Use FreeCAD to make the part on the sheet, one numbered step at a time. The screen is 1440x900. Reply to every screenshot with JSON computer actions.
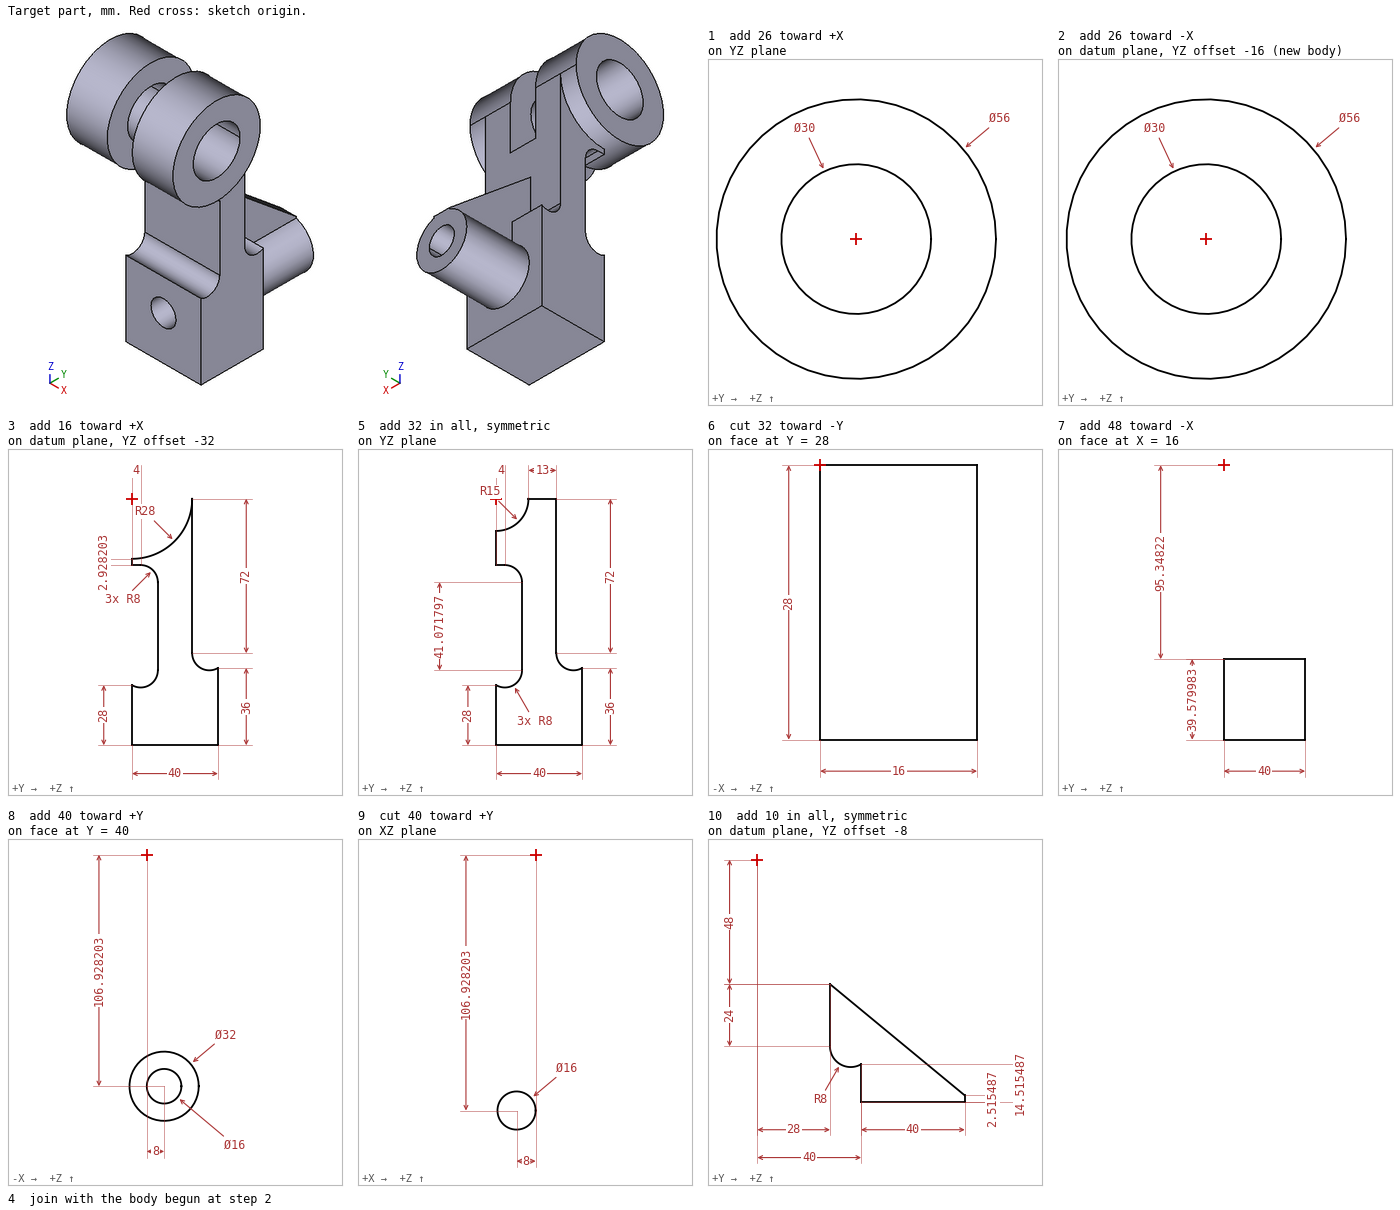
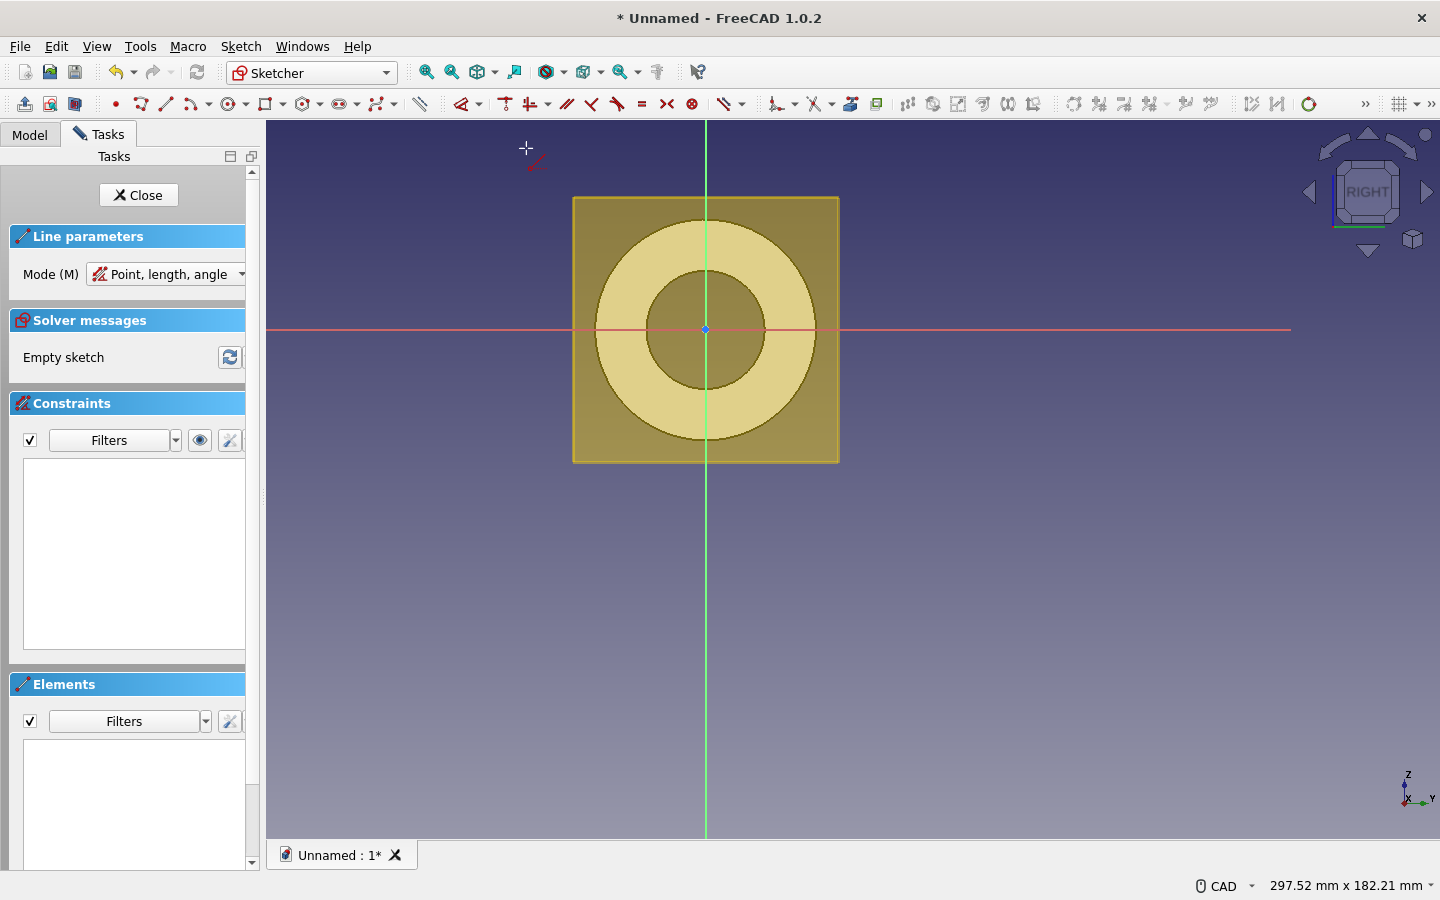
{"action": "left_click", "coordinate": [816, 614]}
{"action": "left_click", "coordinate": [816, 330]}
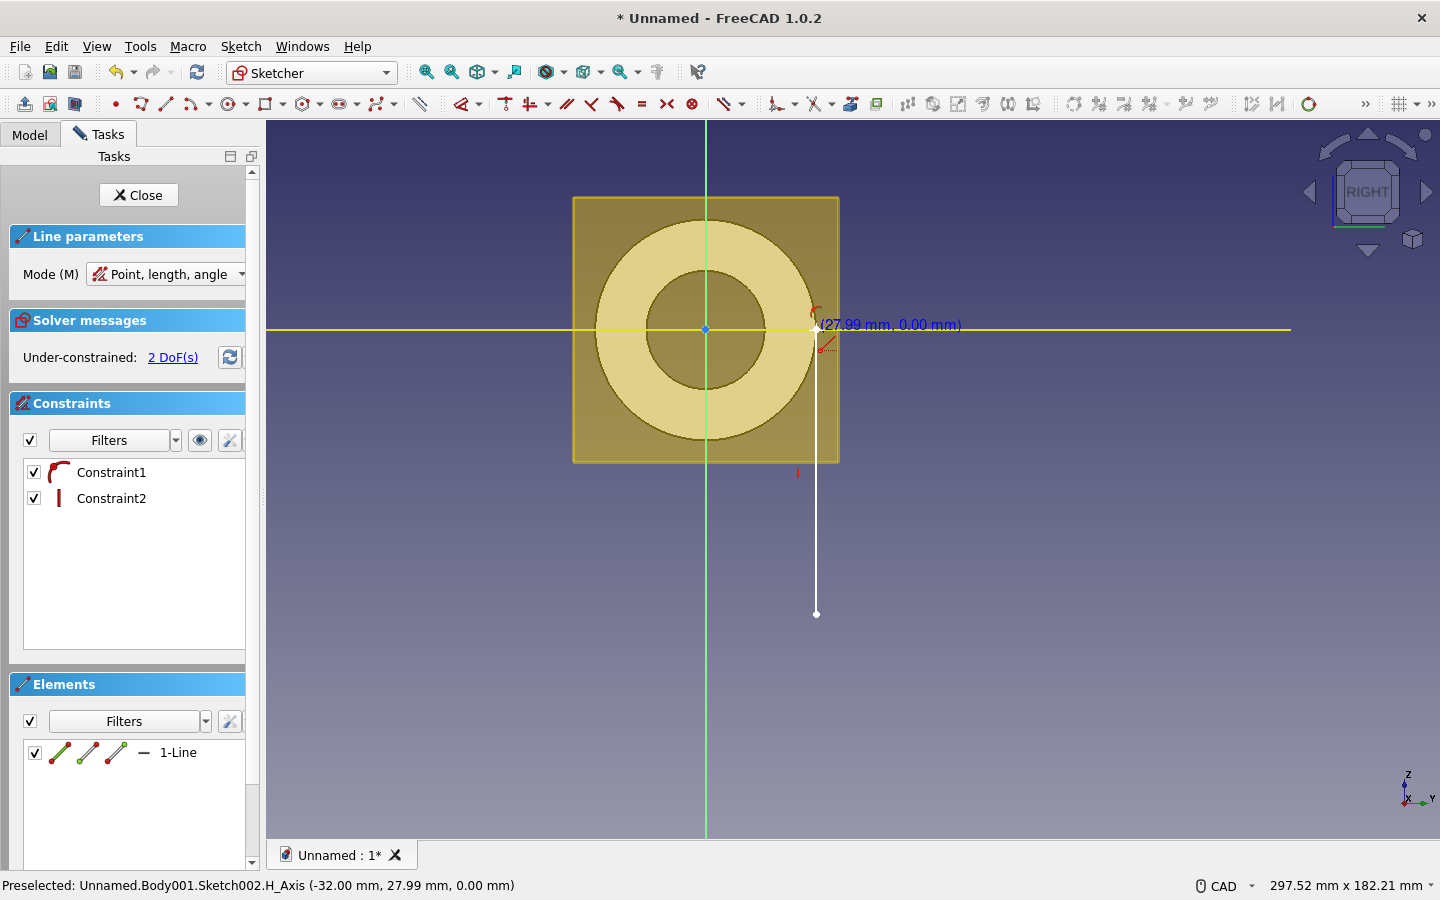
{"action": "left_click", "coordinate": [141, 104]}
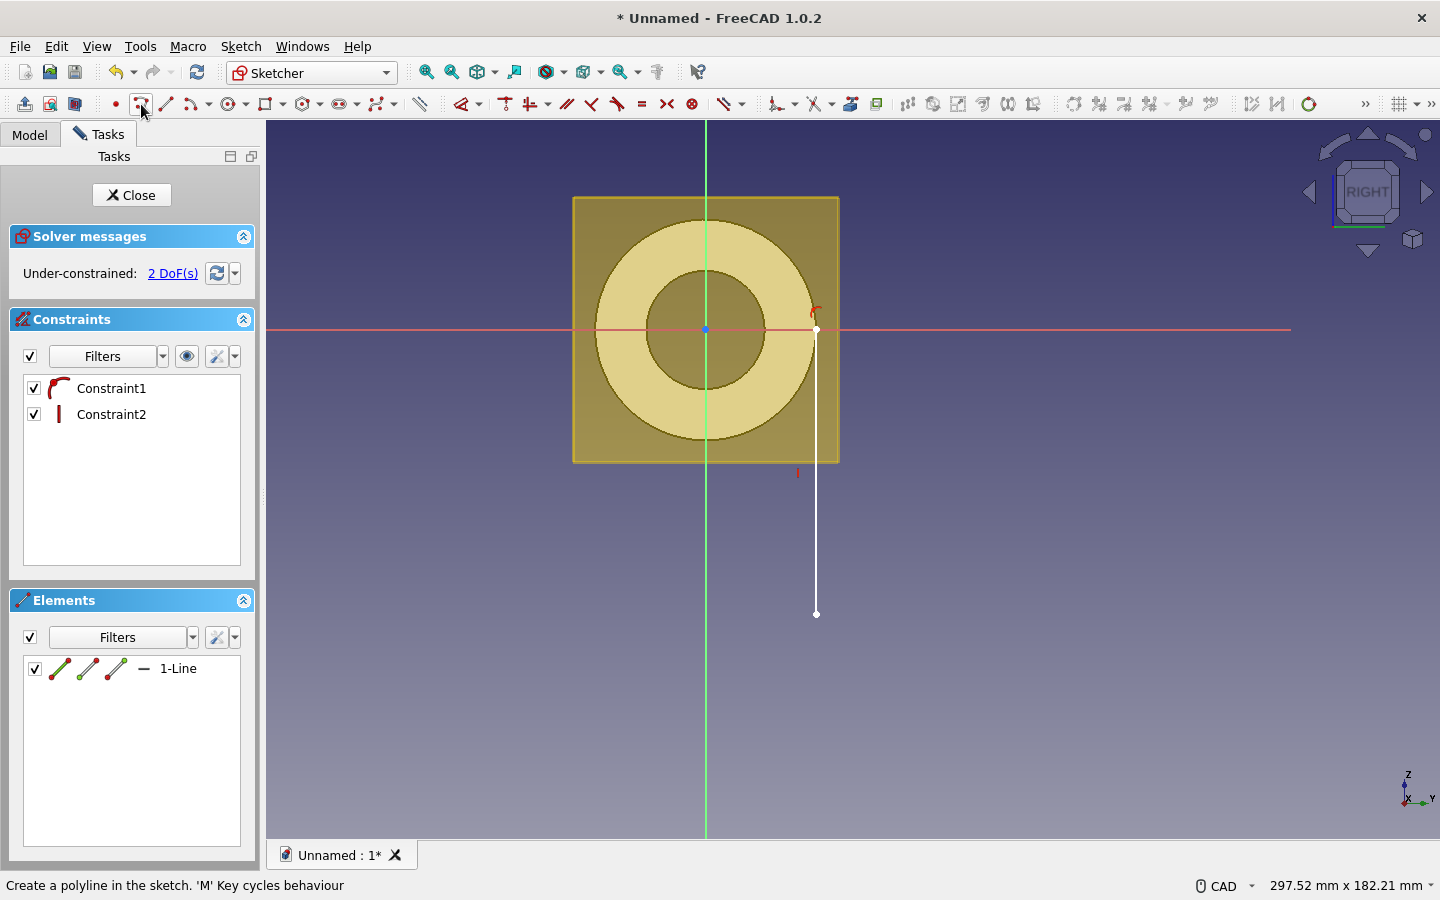
{"action": "left_click", "coordinate": [706, 440]}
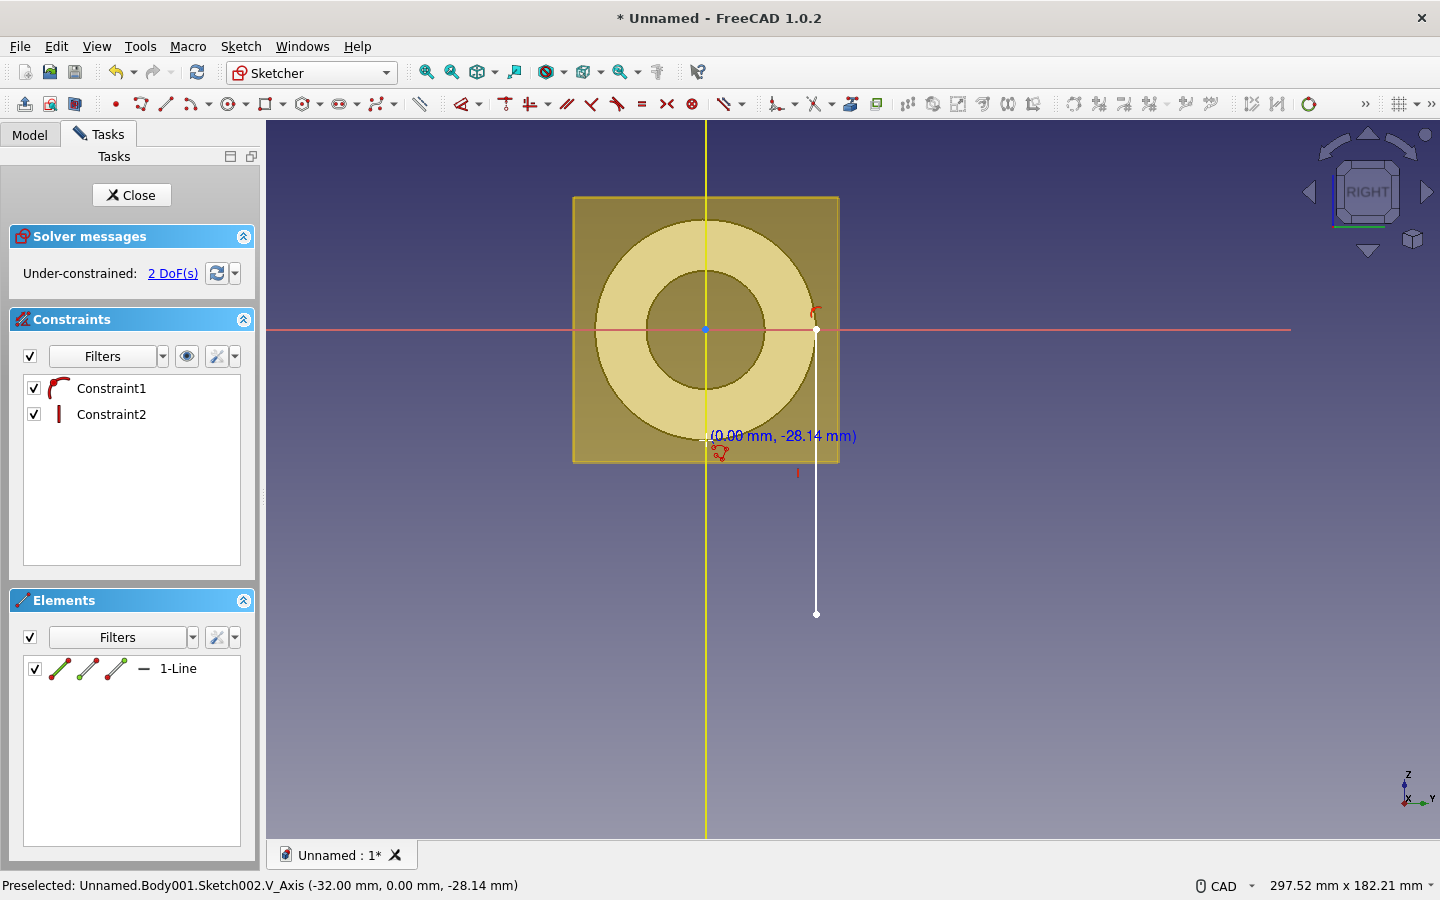
{"action": "scroll", "coordinate": [706, 452], "scroll_direction": "up", "scroll_amount": 2}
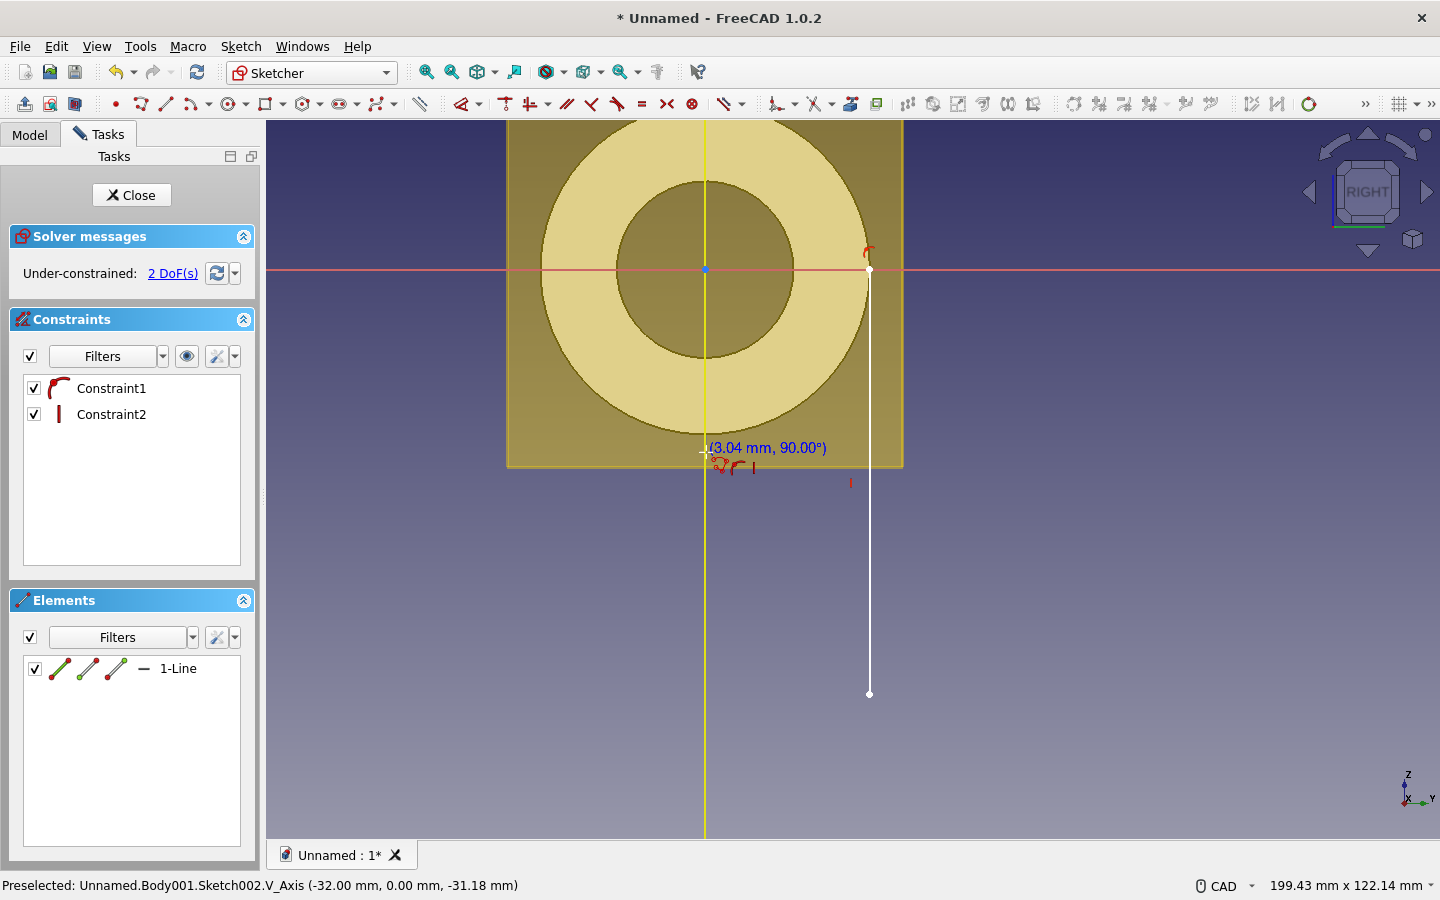
{"action": "left_click", "coordinate": [714, 452]}
{"action": "left_click", "coordinate": [729, 452]}
{"action": "right_click", "coordinate": [729, 452]}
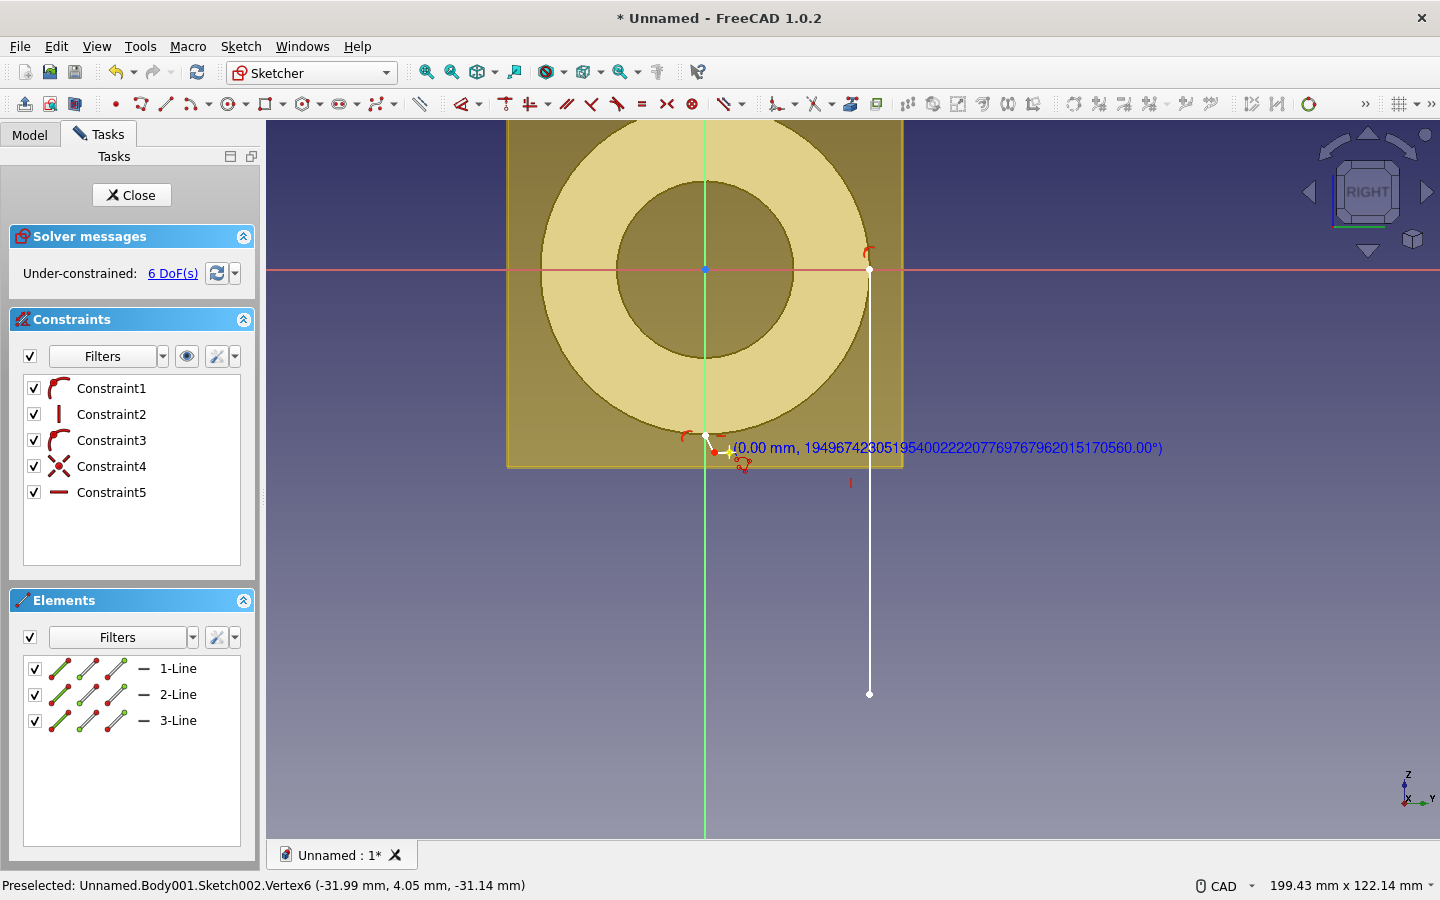
{"action": "left_click", "coordinate": [166, 104]}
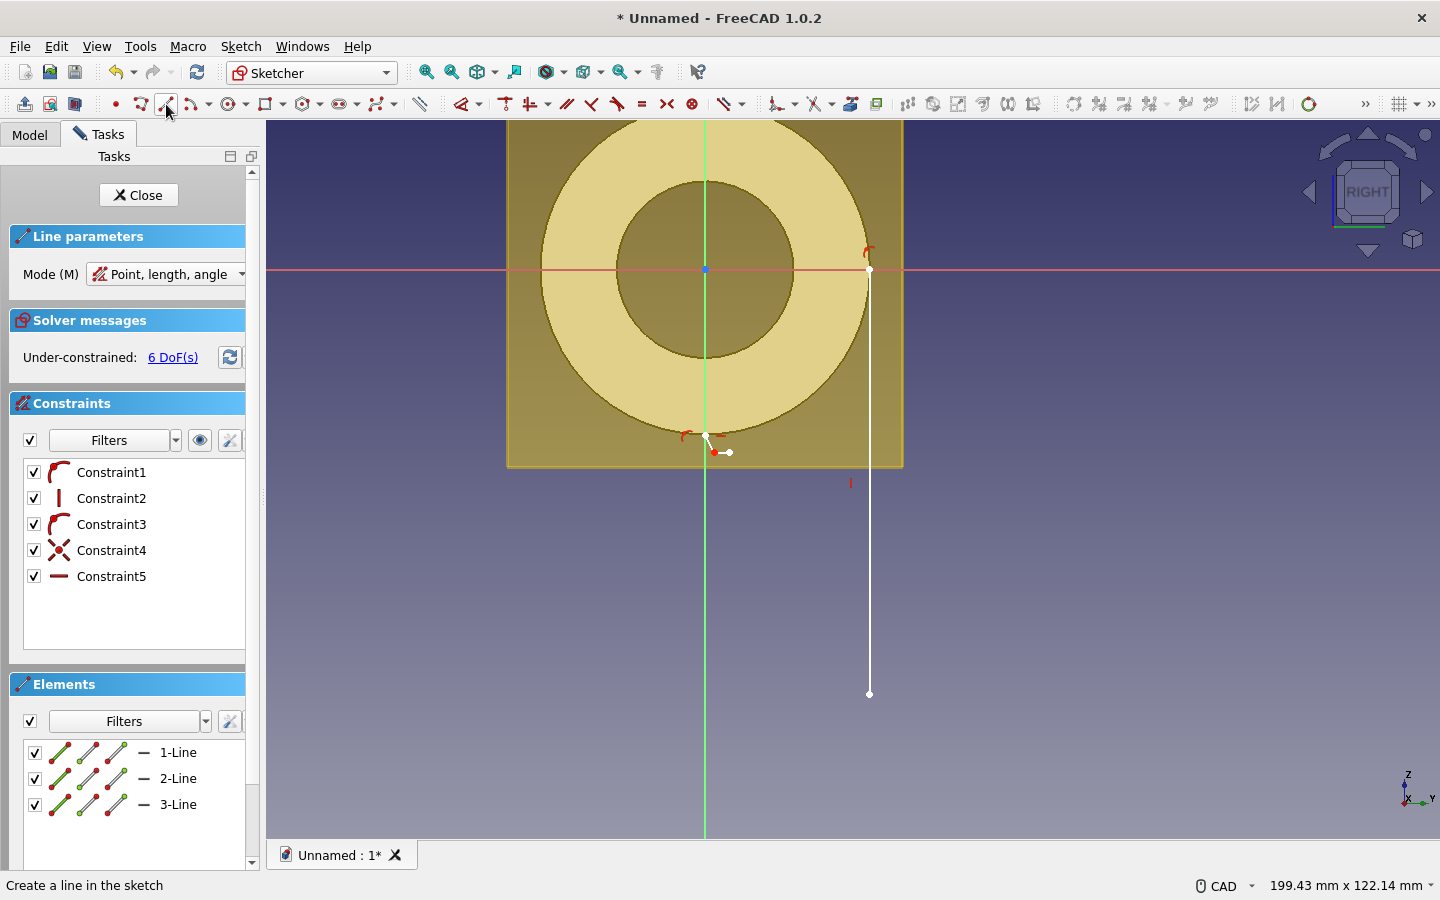
{"action": "left_click", "coordinate": [776, 499]}
{"action": "left_click", "coordinate": [776, 741]}